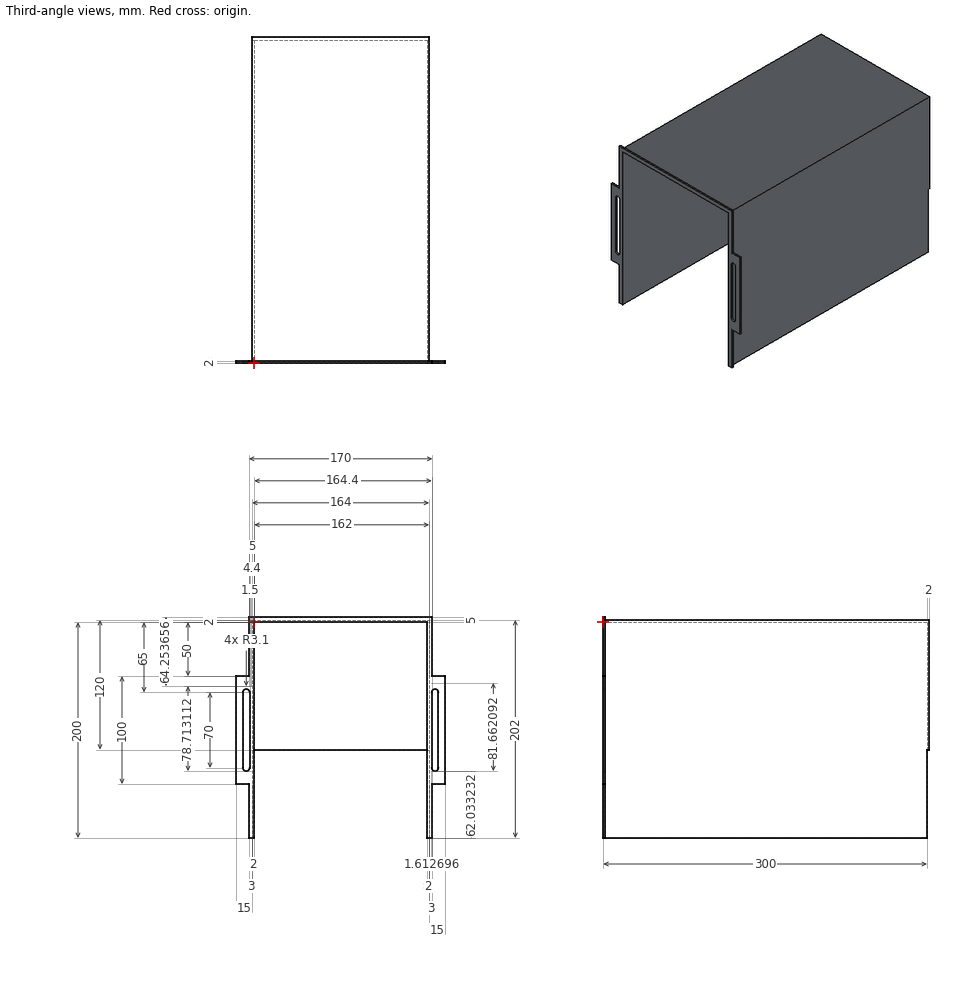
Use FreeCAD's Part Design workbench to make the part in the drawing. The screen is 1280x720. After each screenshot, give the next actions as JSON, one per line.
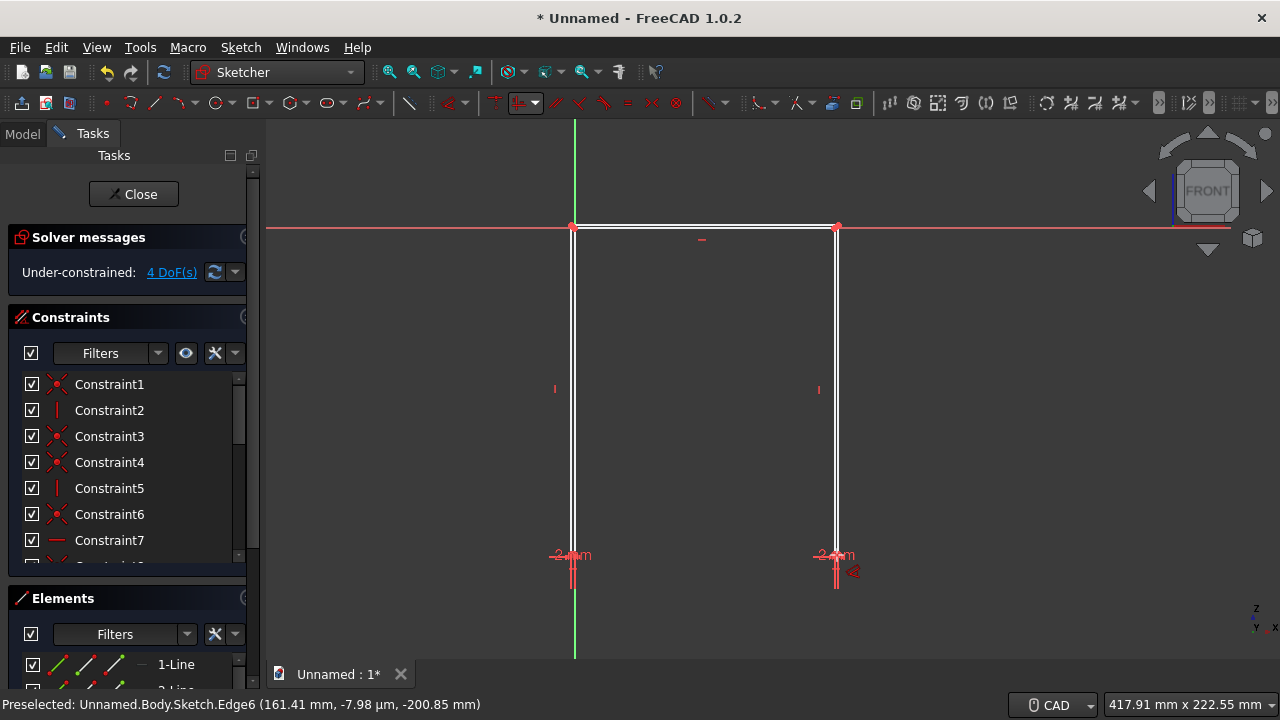
{"action": "scroll", "coordinate": [571, 225], "scroll_direction": "up", "scroll_amount": 13}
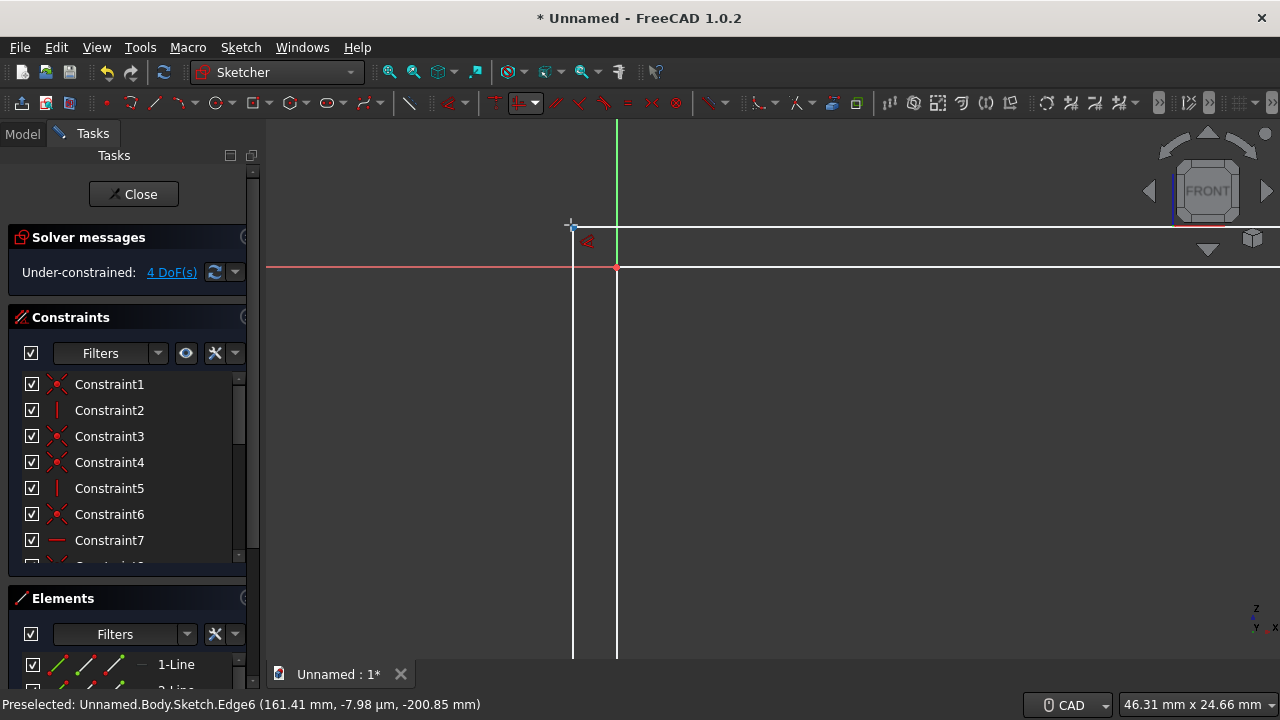
{"action": "left_click", "coordinate": [573, 227]}
{"action": "left_click", "coordinate": [539, 247]}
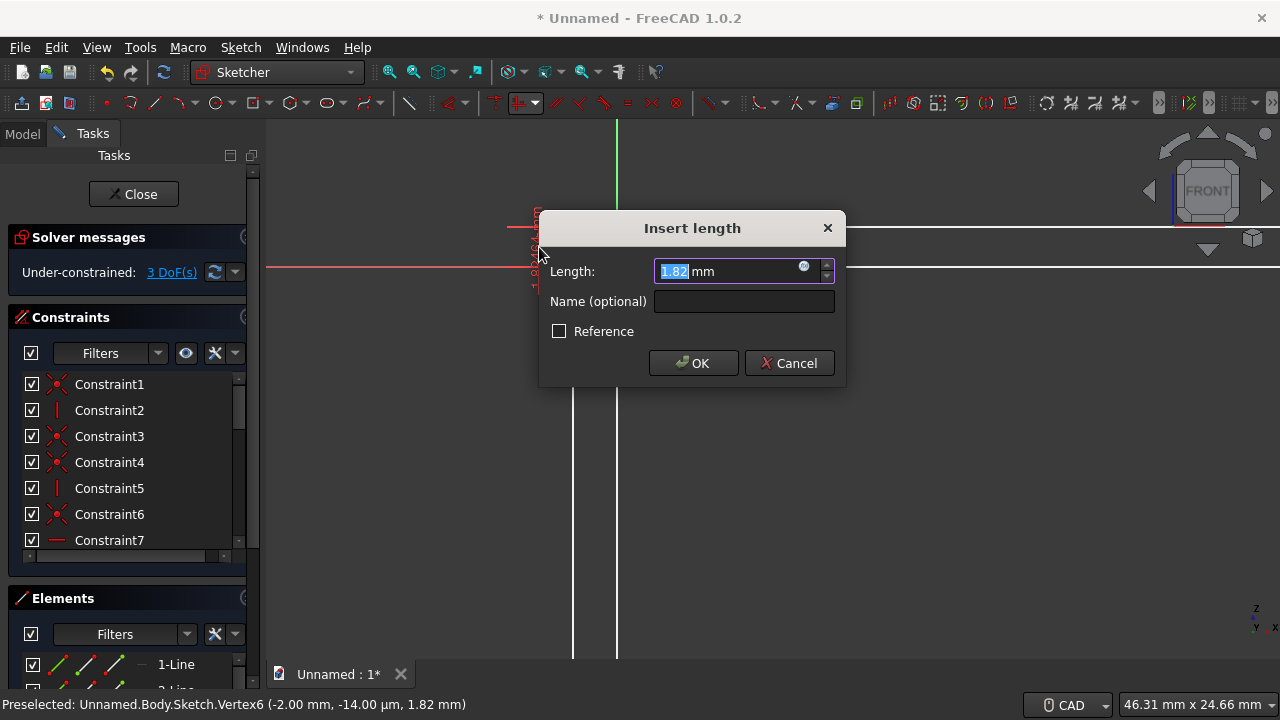
{"action": "type", "text": "2"}
{"action": "key", "text": "Return"}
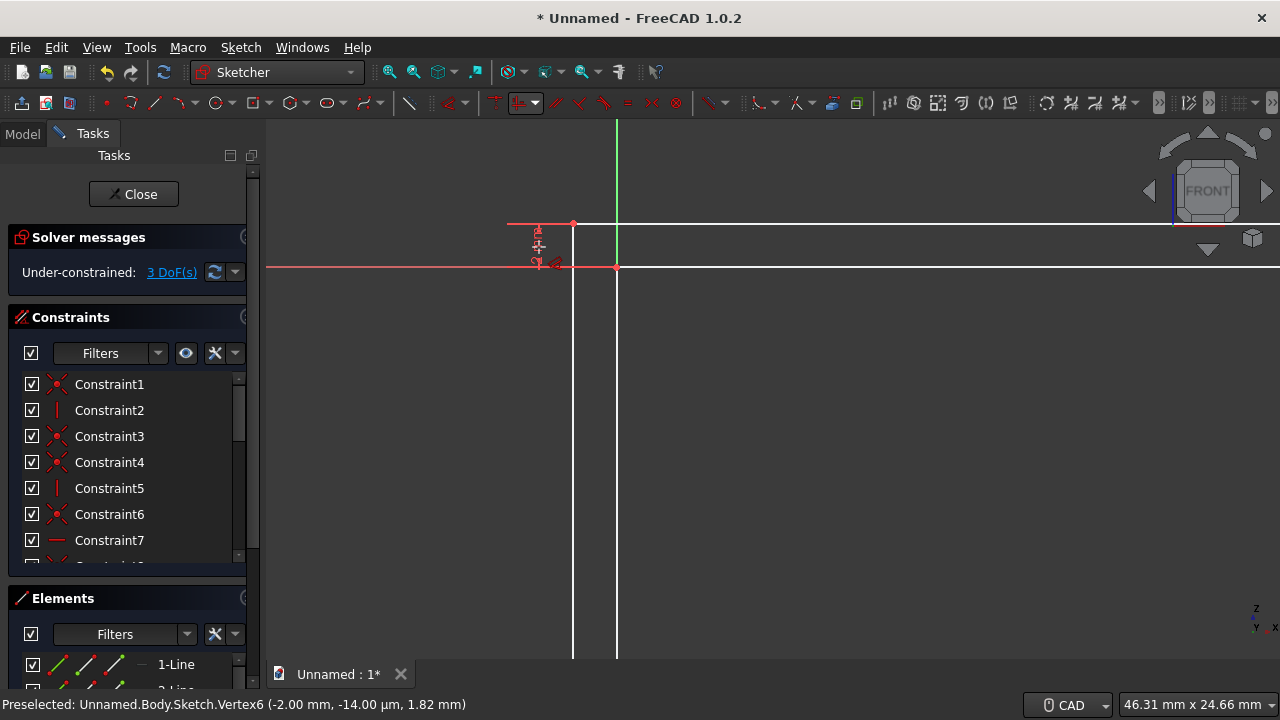
{"action": "scroll", "coordinate": [571, 225], "scroll_direction": "down", "scroll_amount": 13}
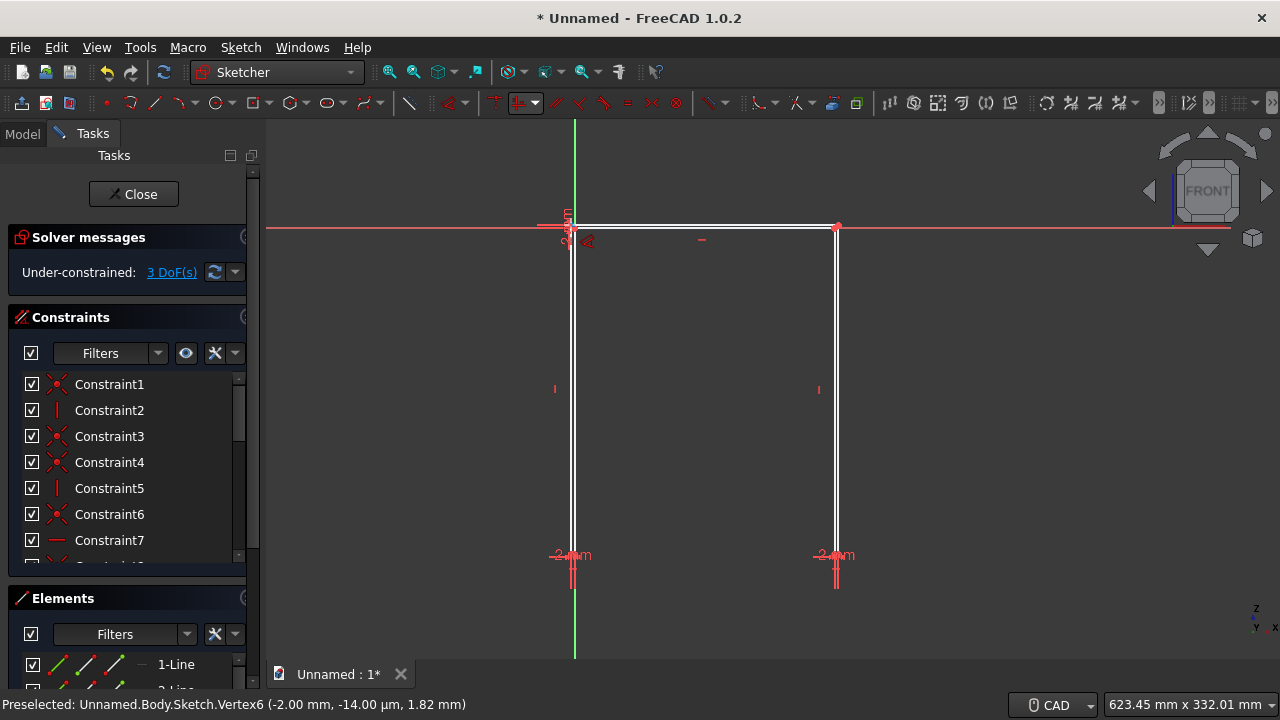
{"action": "scroll", "coordinate": [575, 326], "scroll_direction": "up", "scroll_amount": 8}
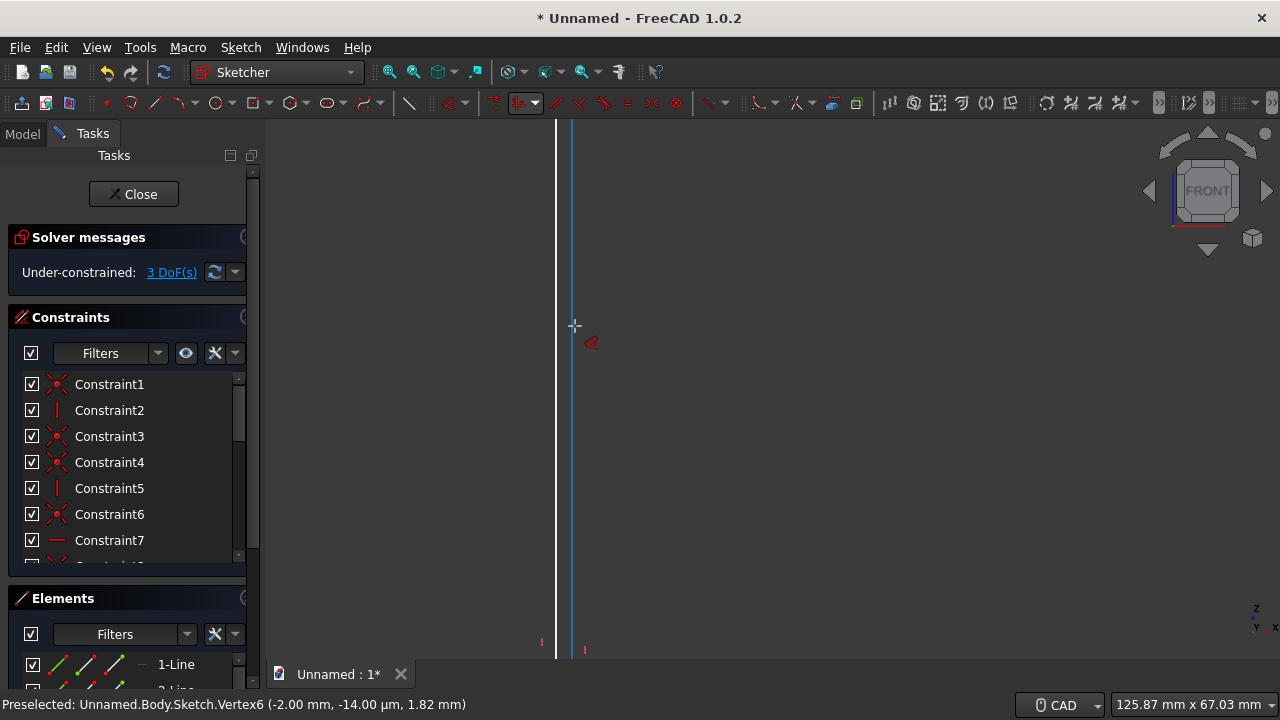
{"action": "left_click", "coordinate": [572, 326]}
{"action": "left_click", "coordinate": [538, 389]}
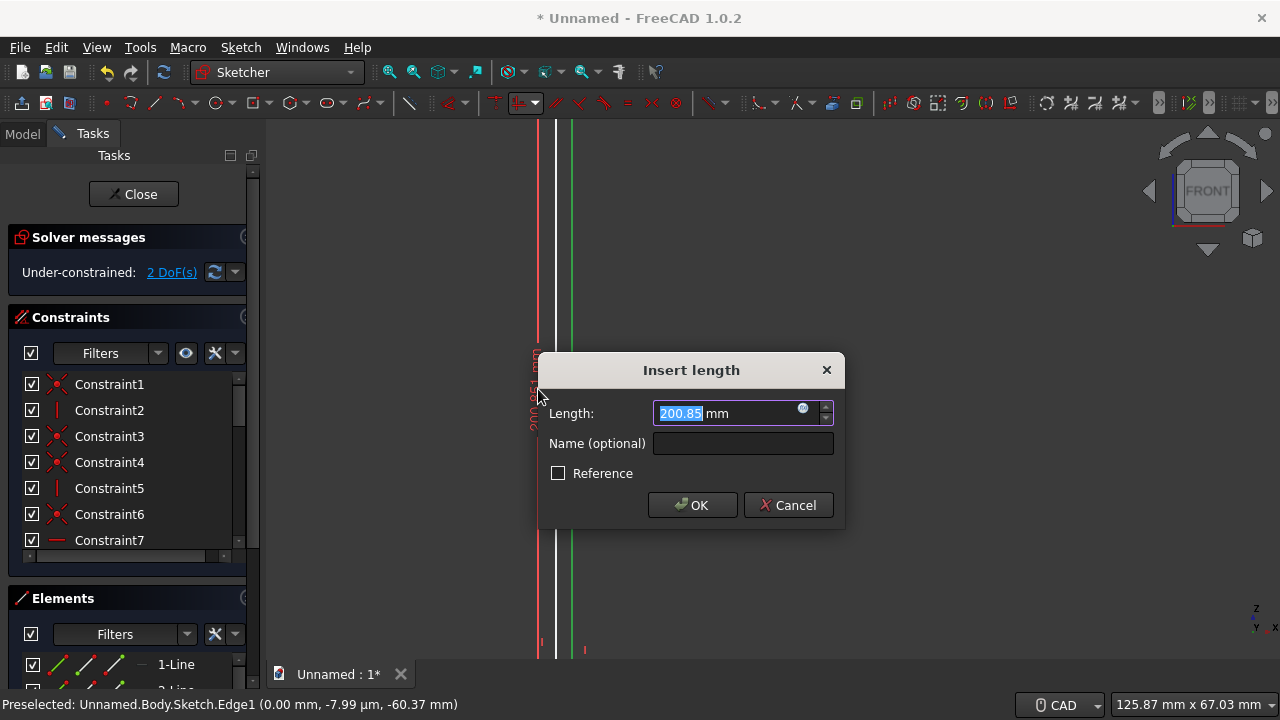
{"action": "type", "text": "200"}
{"action": "key", "text": "Return"}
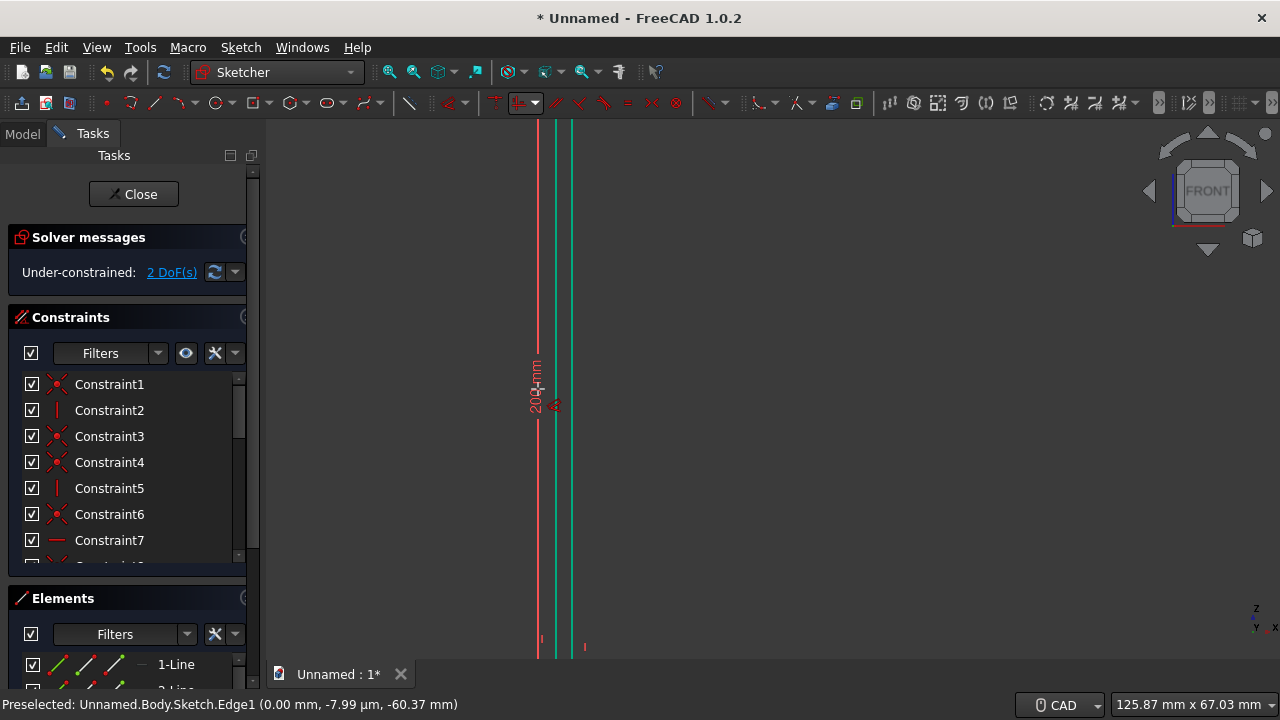
{"action": "scroll", "coordinate": [575, 326], "scroll_direction": "down", "scroll_amount": 8}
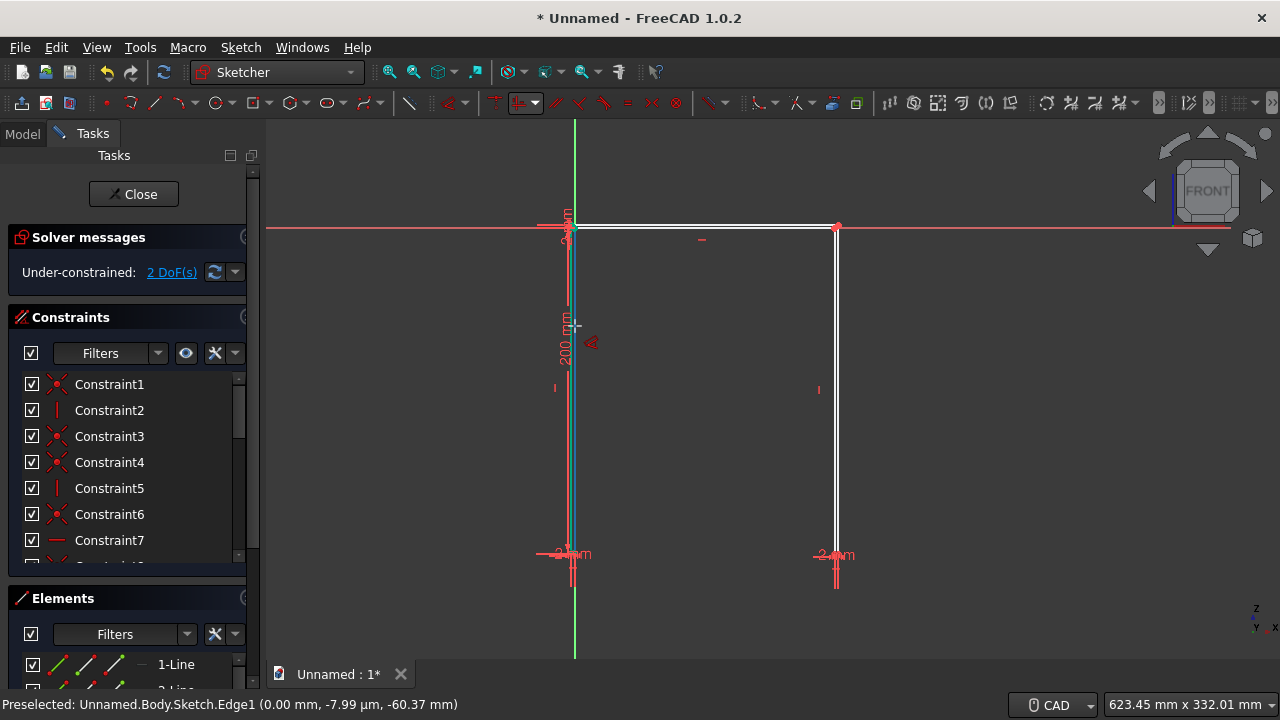
{"action": "scroll", "coordinate": [651, 225], "scroll_direction": "up", "scroll_amount": 8}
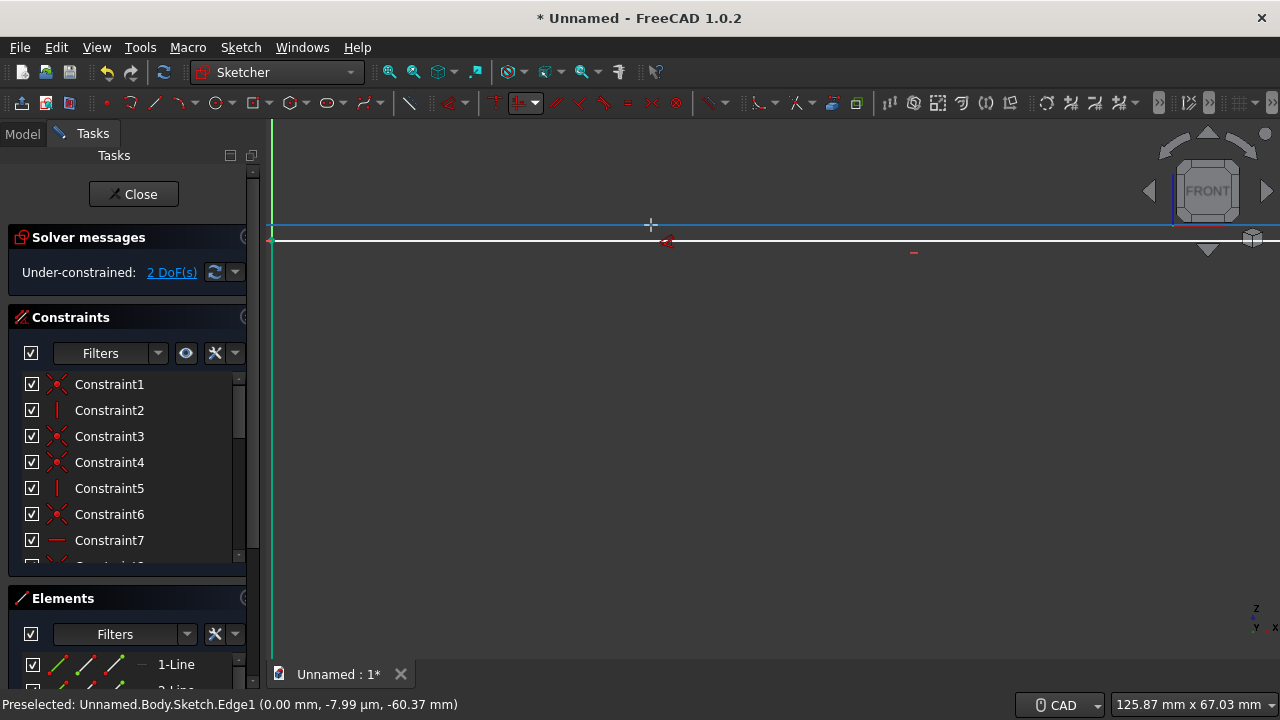
{"action": "left_click", "coordinate": [652, 225]}
{"action": "left_click", "coordinate": [704, 191]}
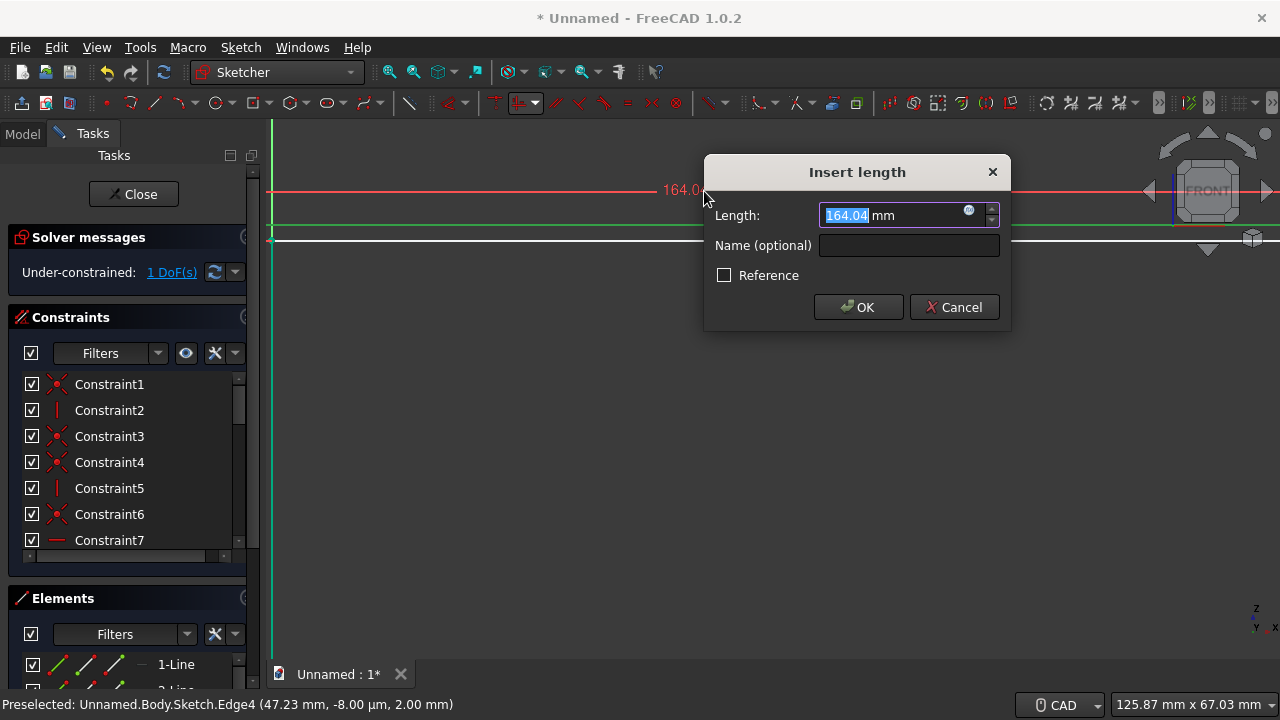
{"action": "type", "text": "164"}
{"action": "key", "text": "Return"}